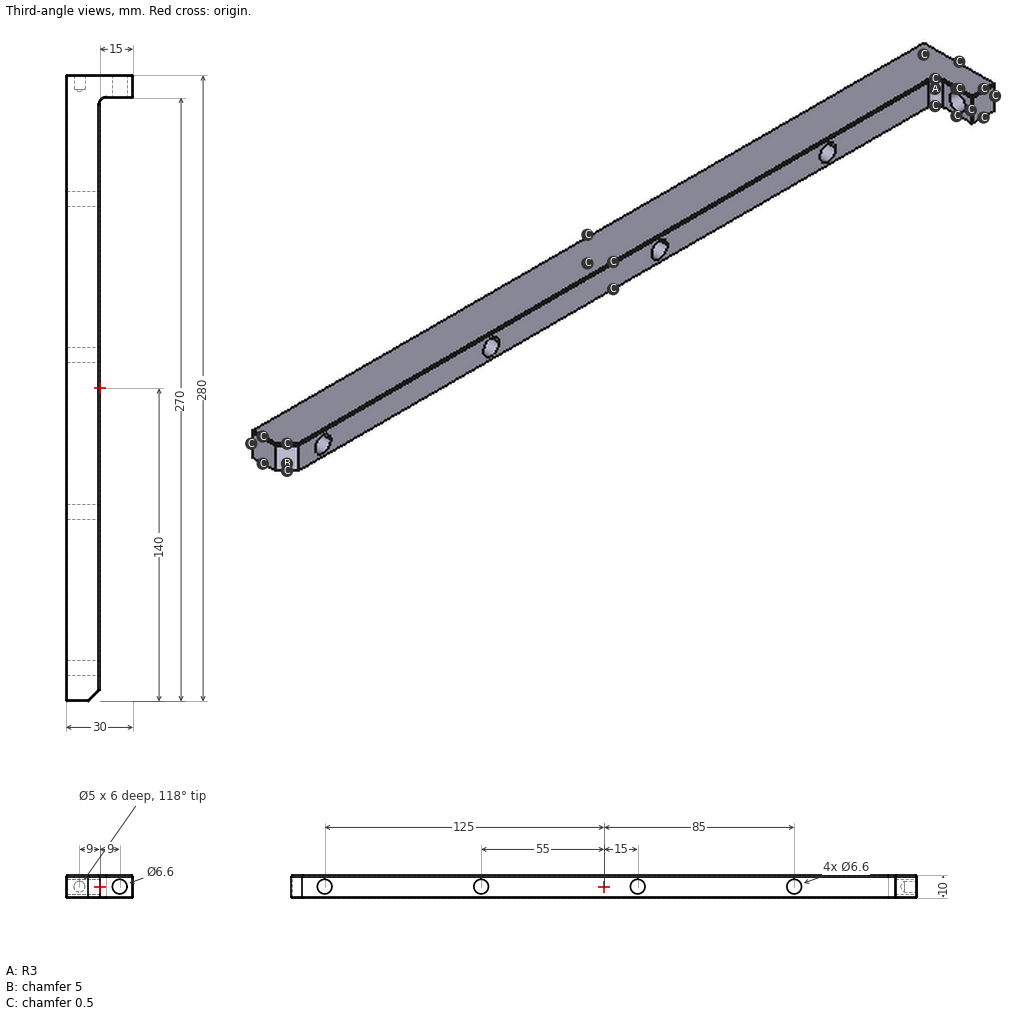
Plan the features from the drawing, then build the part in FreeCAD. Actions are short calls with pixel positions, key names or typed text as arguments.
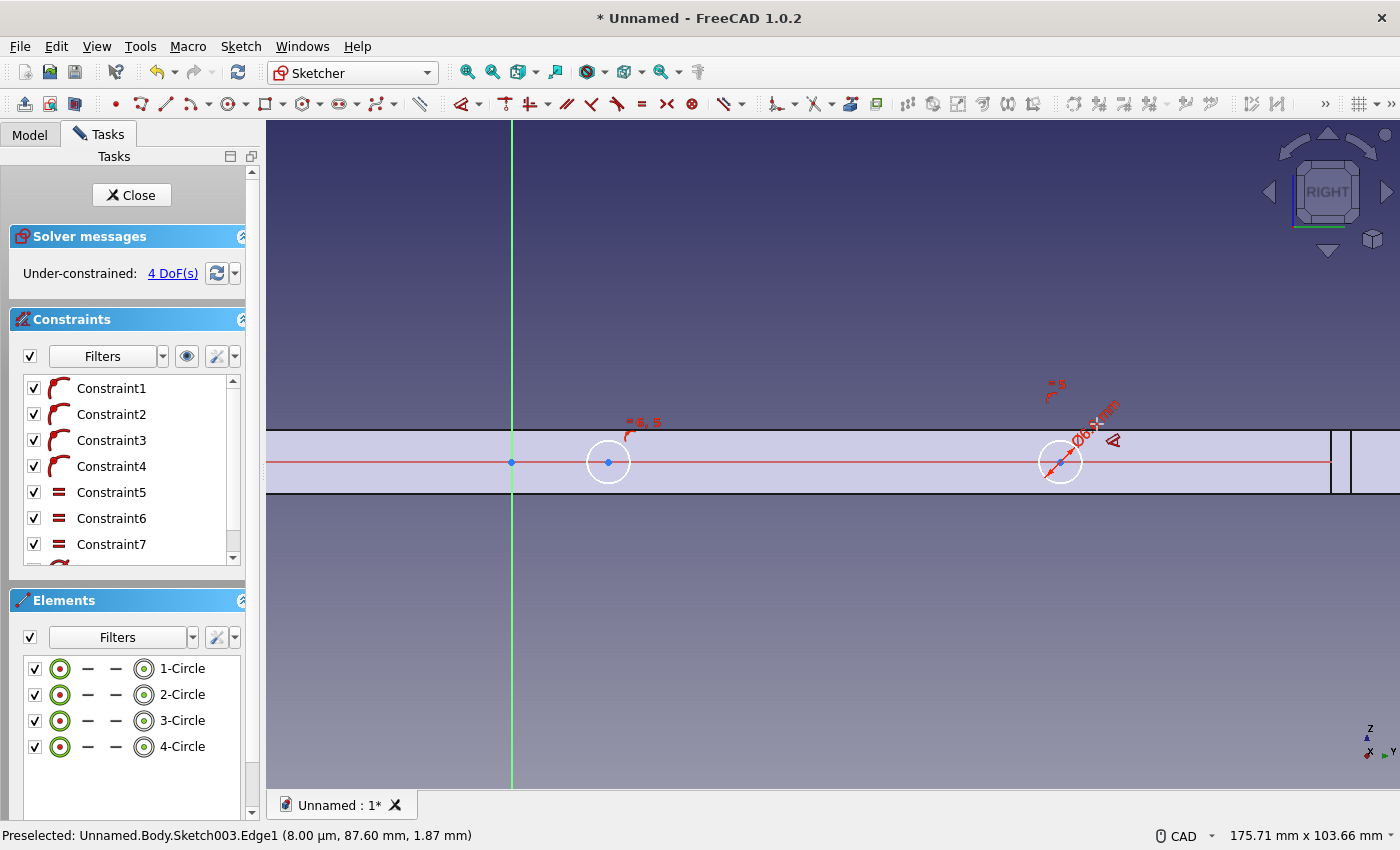
click(1060, 462)
click(786, 496)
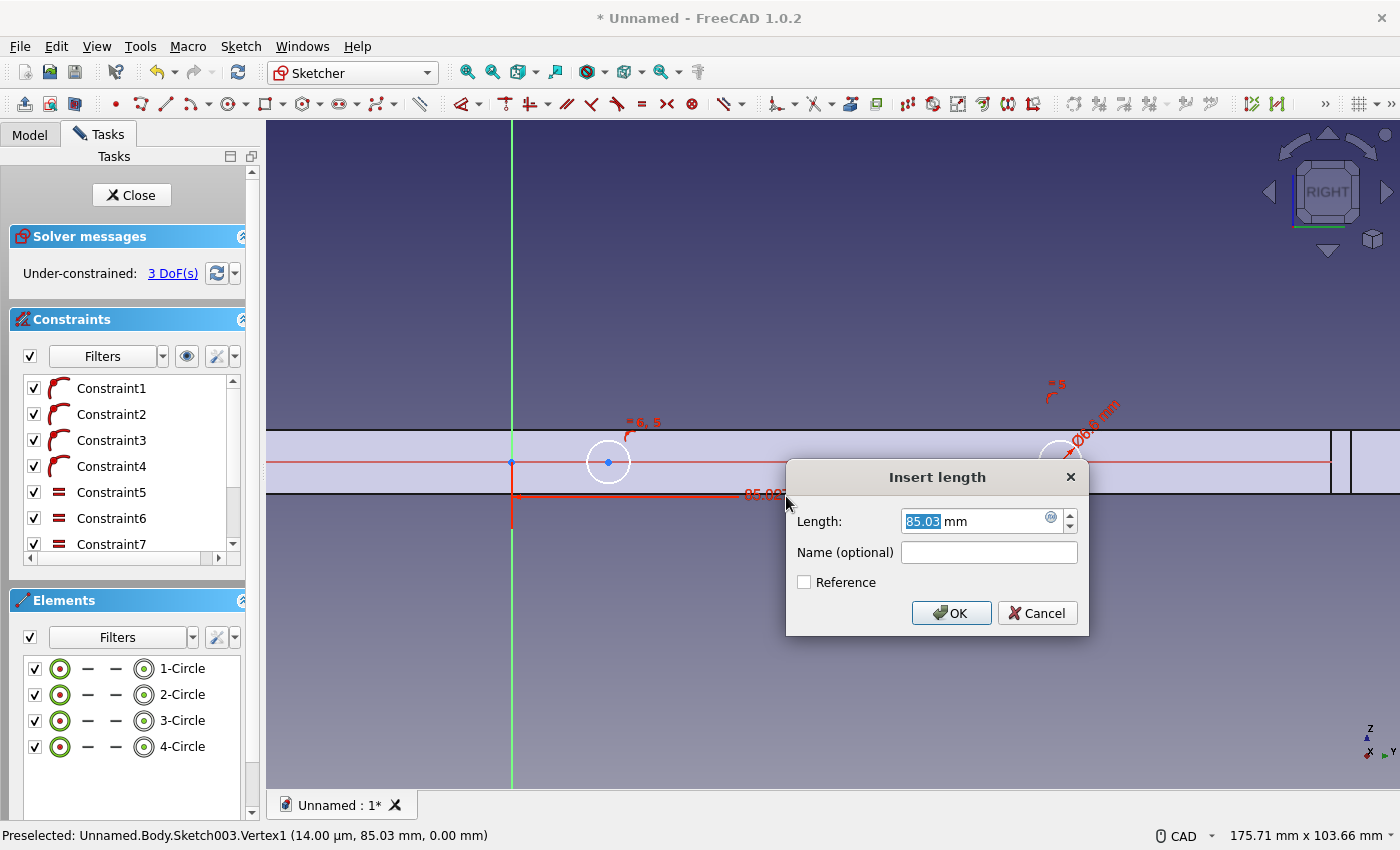
text(85)
key(Return)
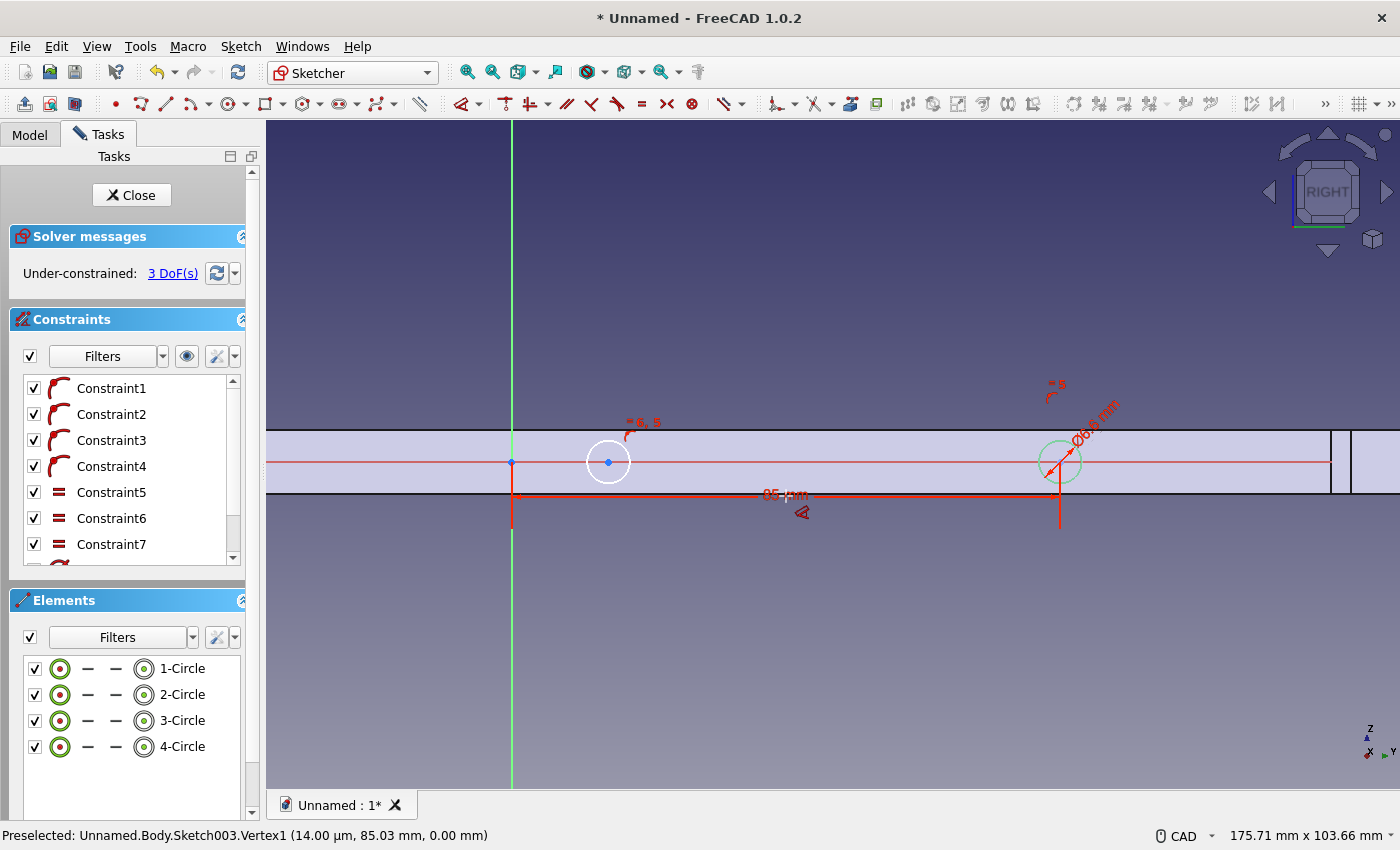
click(609, 462)
click(560, 496)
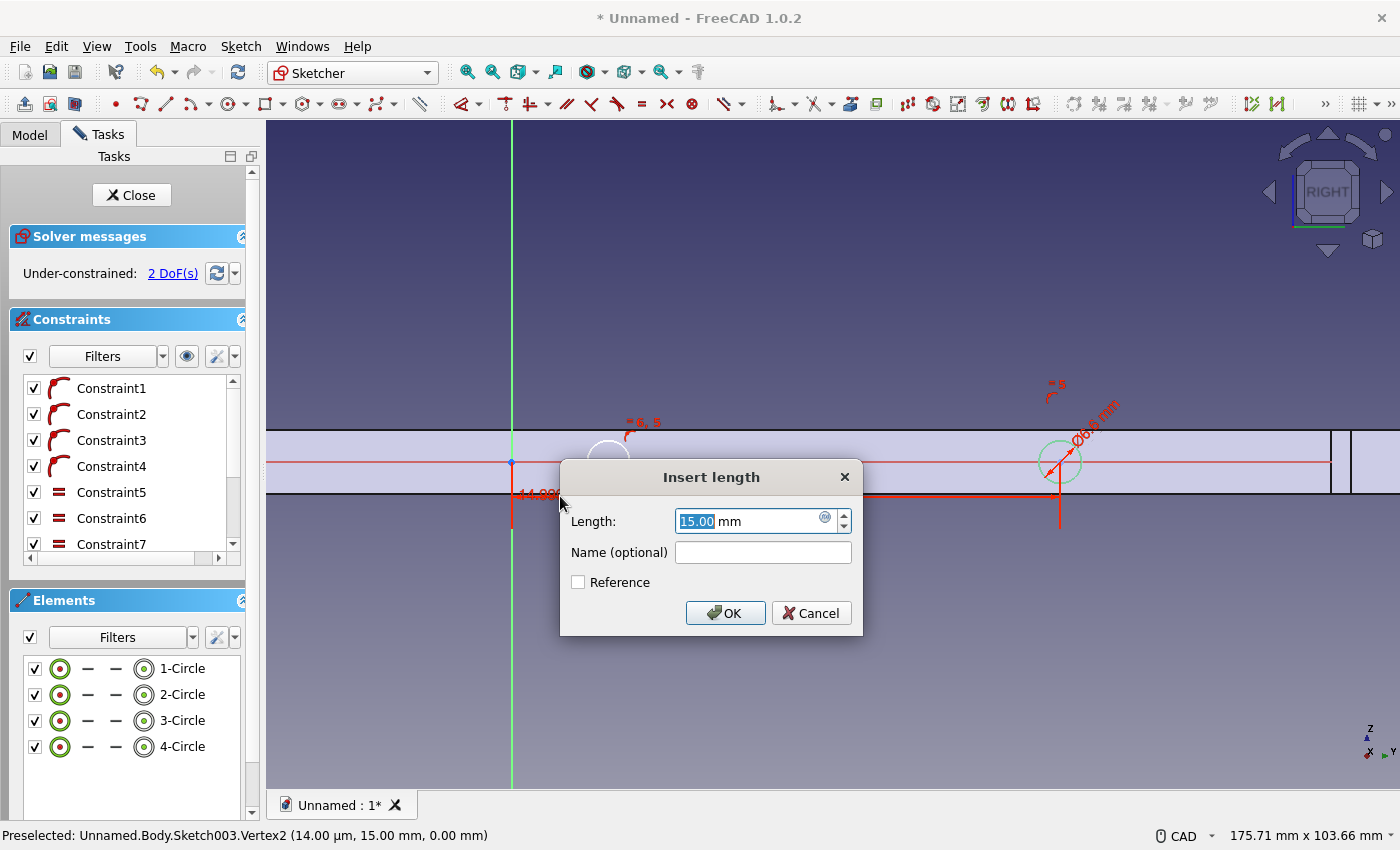
text(15)
key(Return)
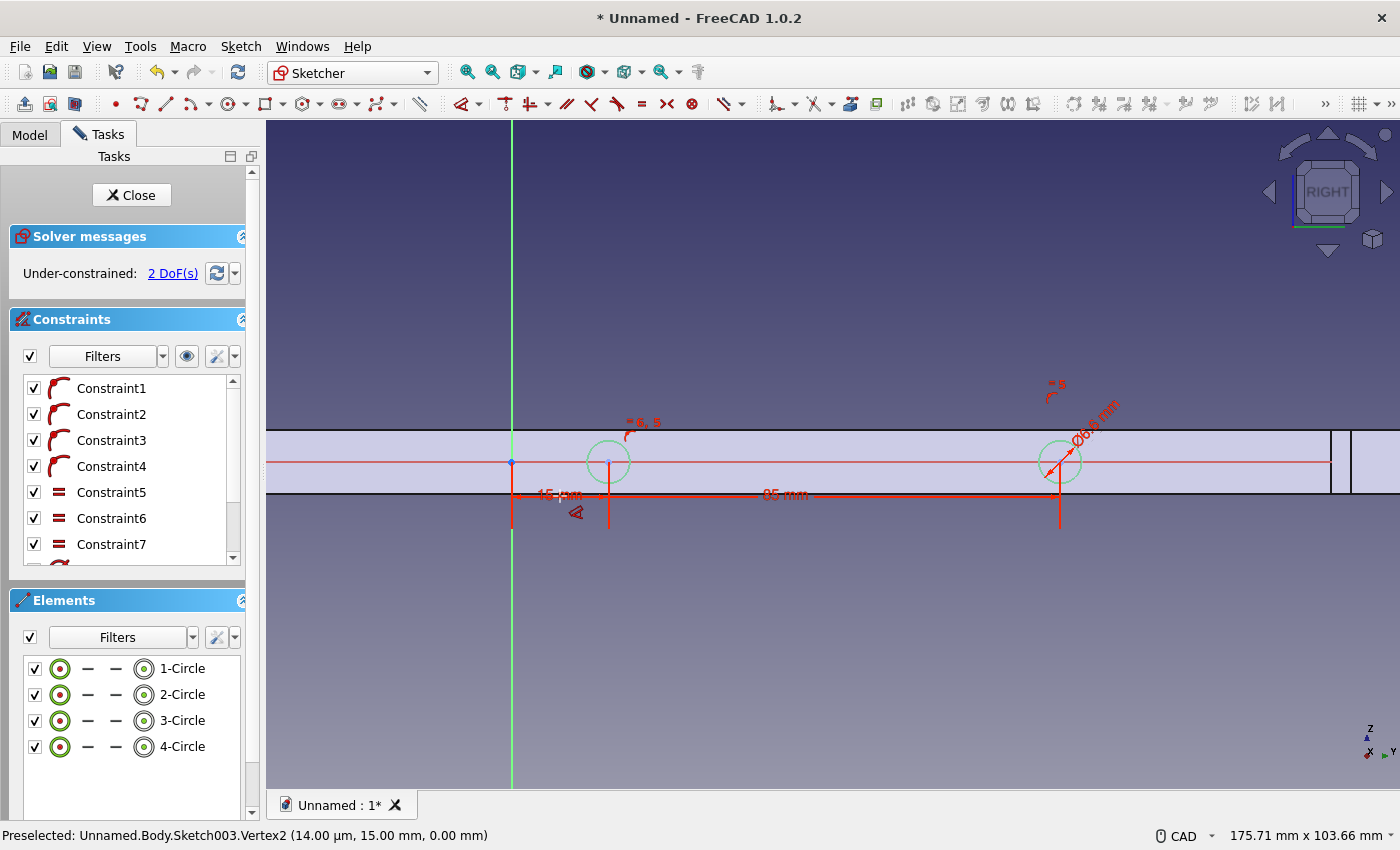
scroll(1076, 448, down, 4)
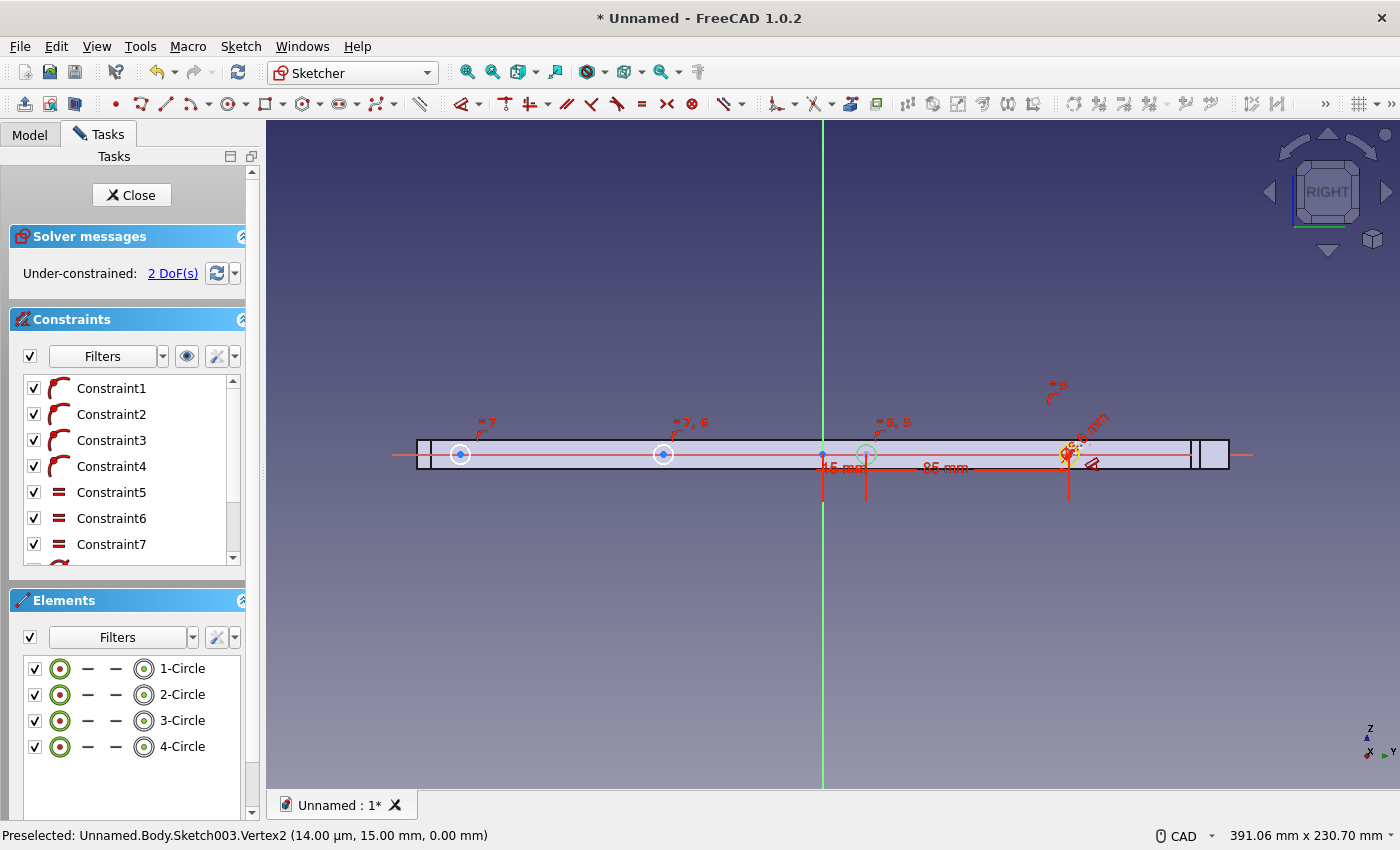
click(664, 455)
click(743, 489)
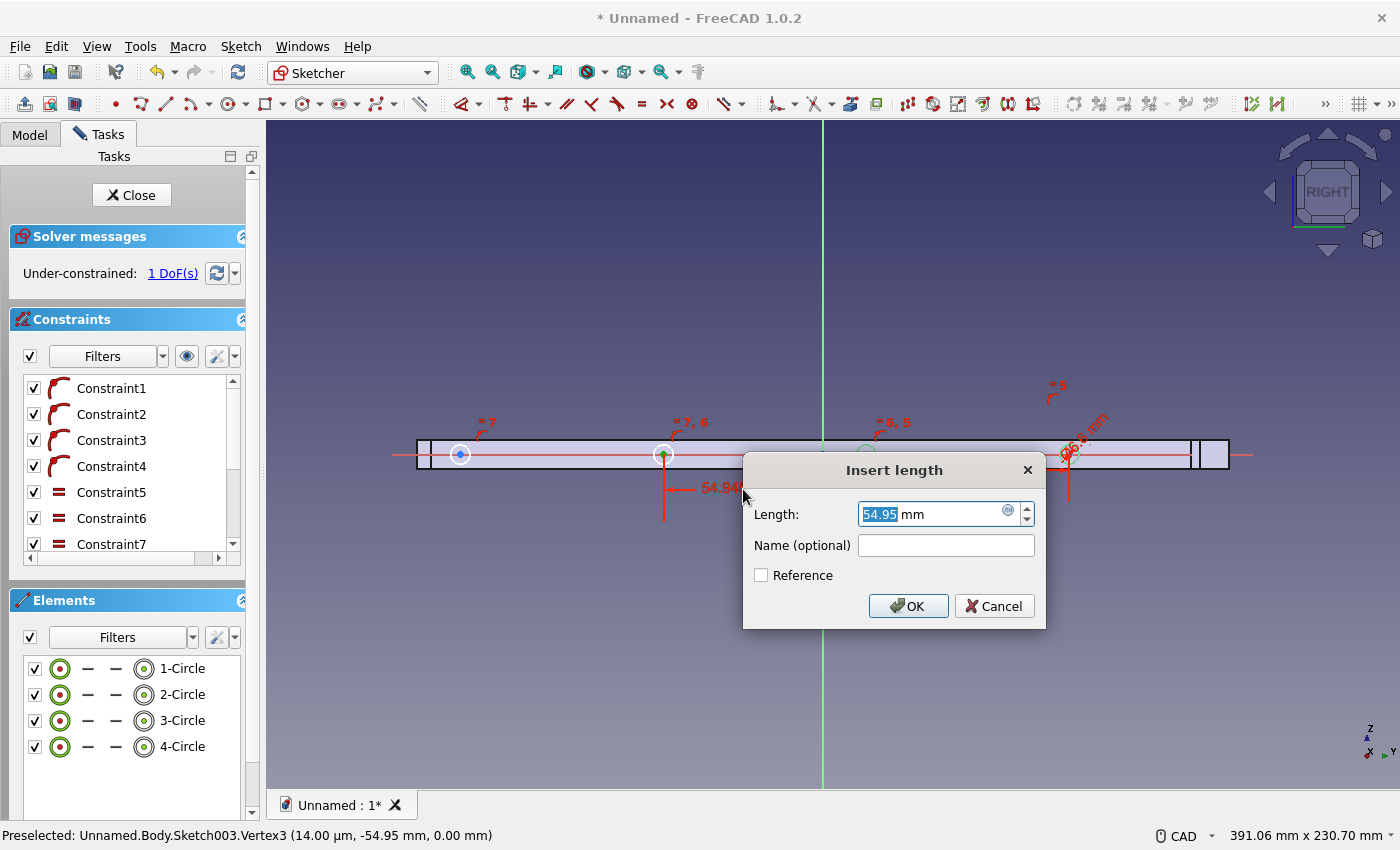
text(55)
key(Return)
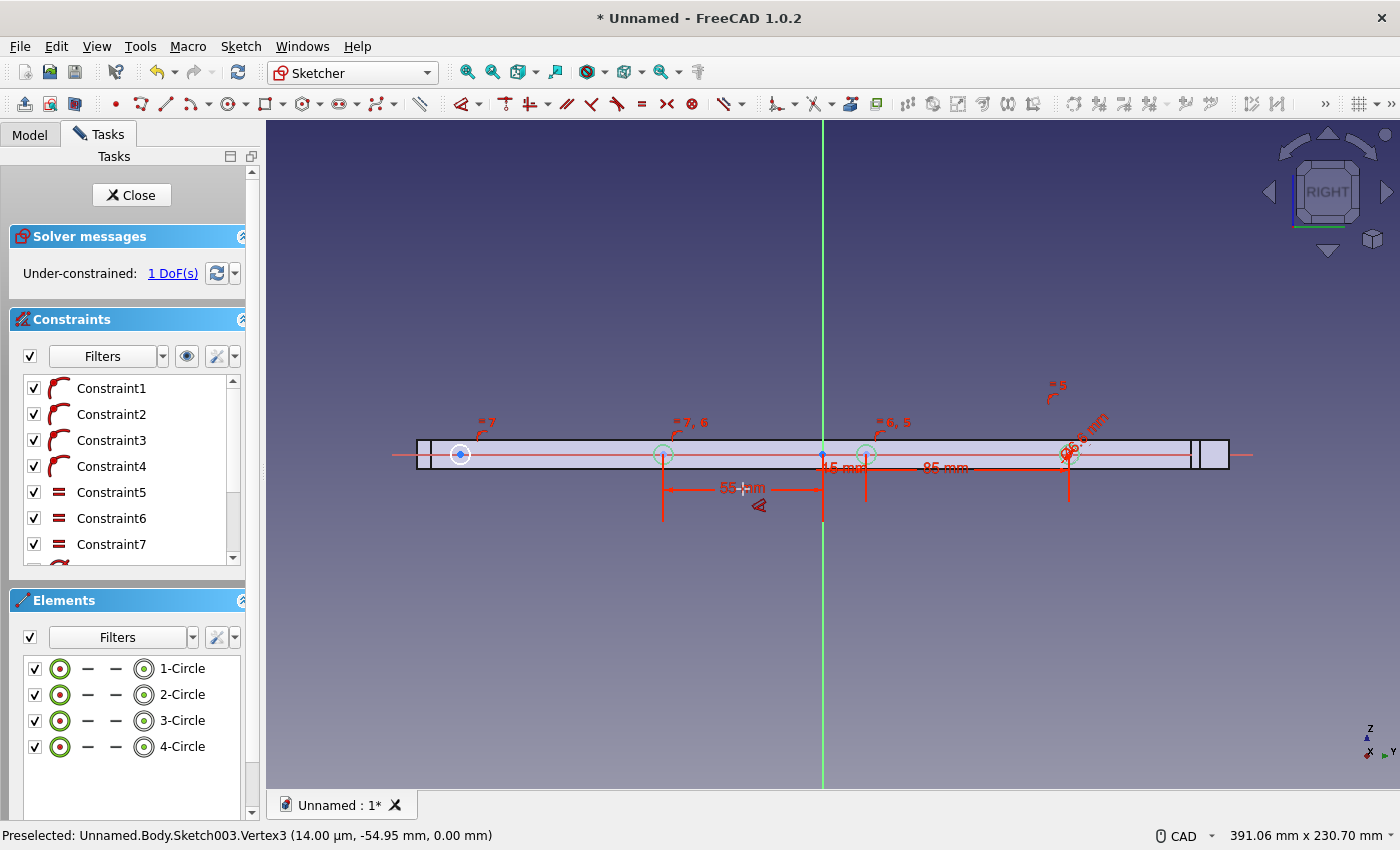
click(460, 455)
click(642, 489)